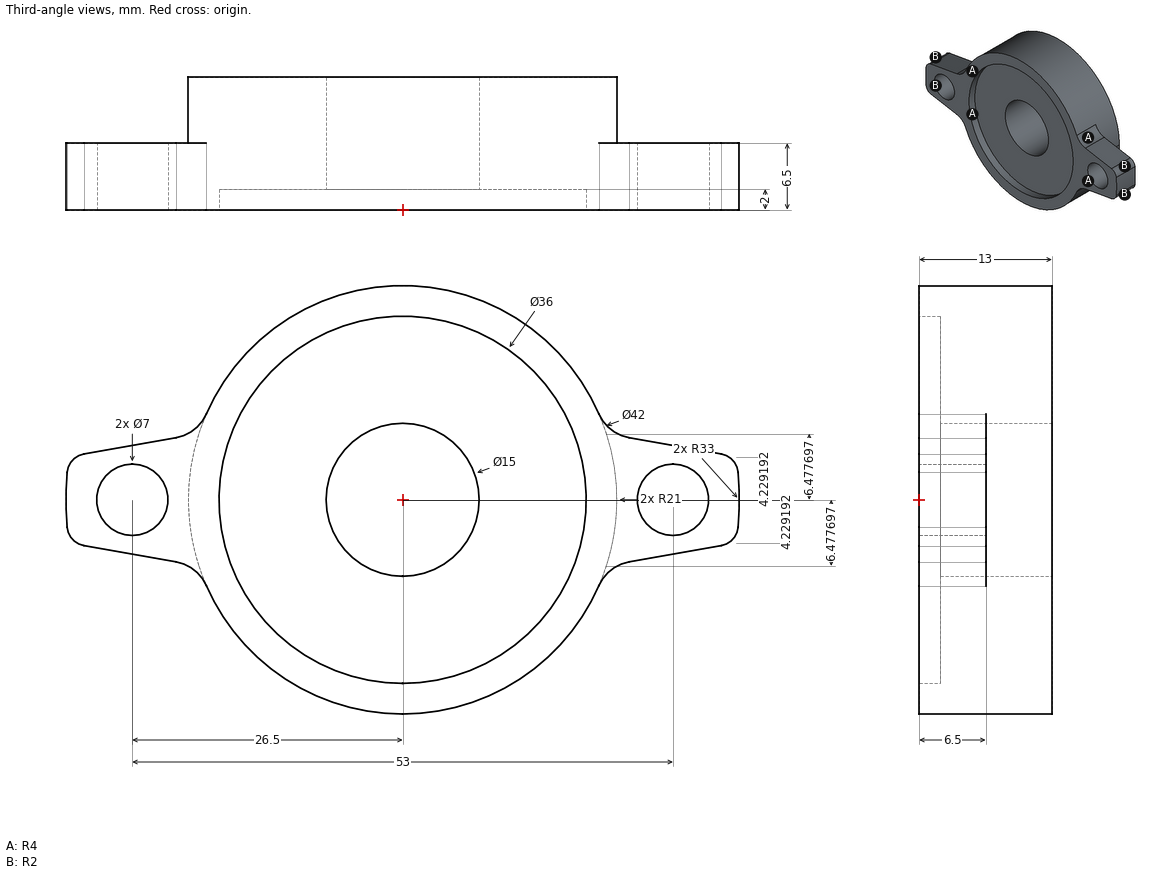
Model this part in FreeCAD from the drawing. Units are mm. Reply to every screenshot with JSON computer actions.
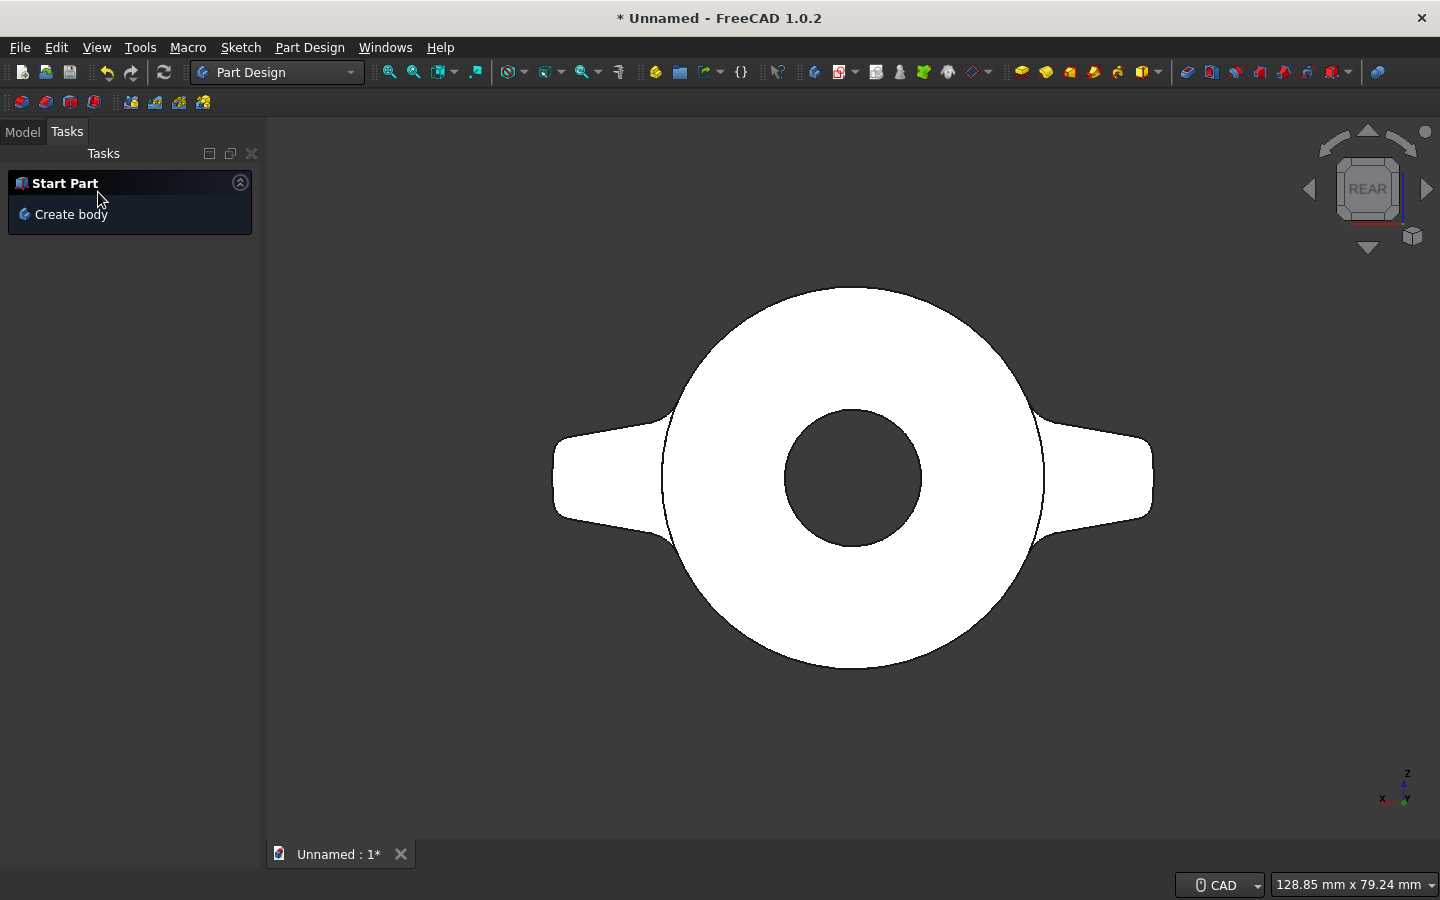
{"action": "left_click", "coordinate": [615, 477]}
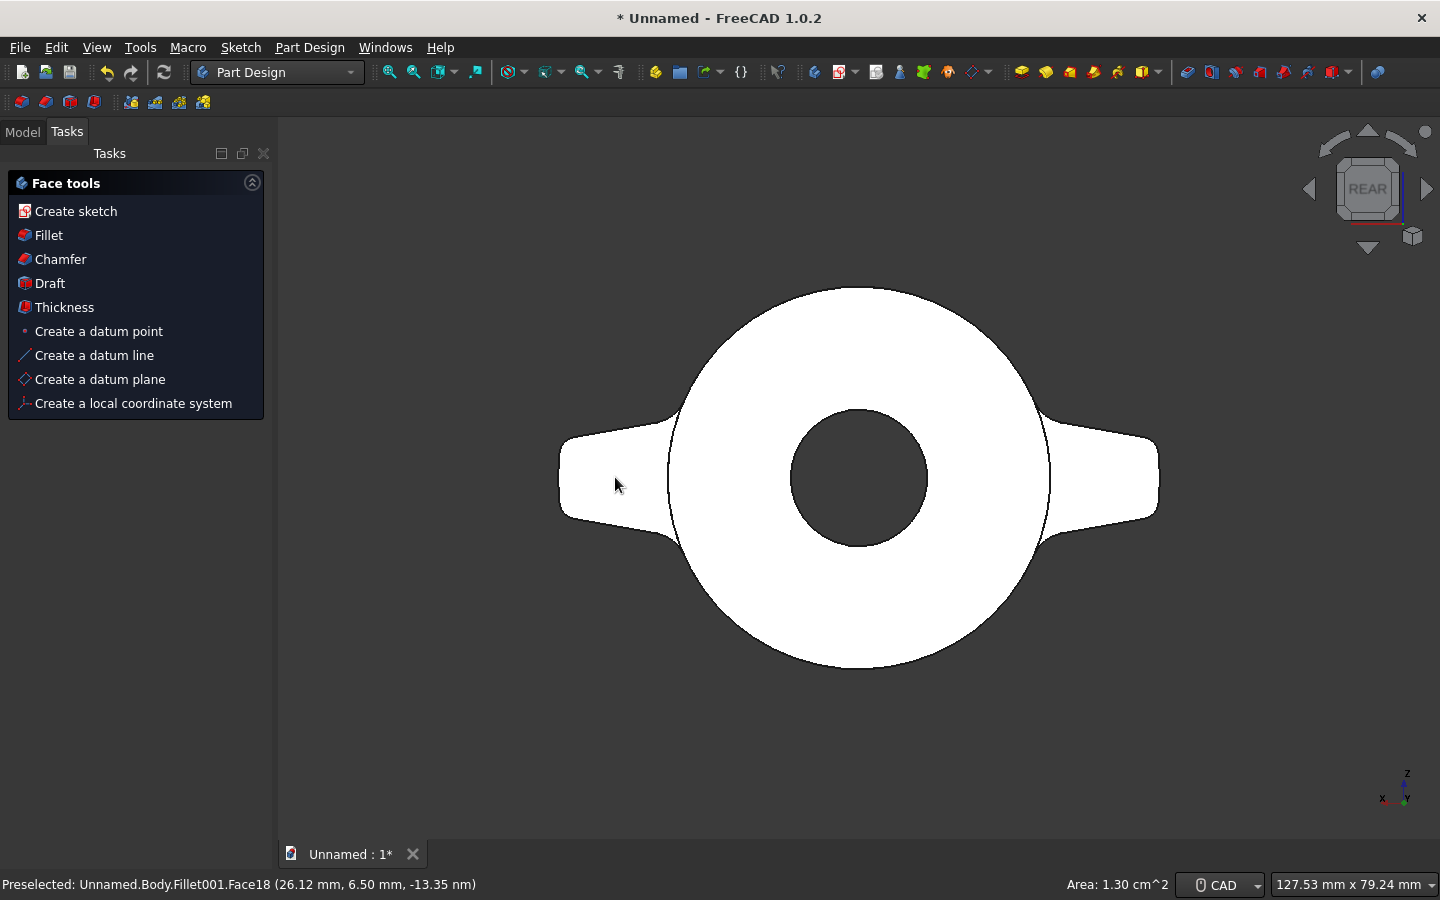
{"action": "left_click", "coordinate": [840, 72]}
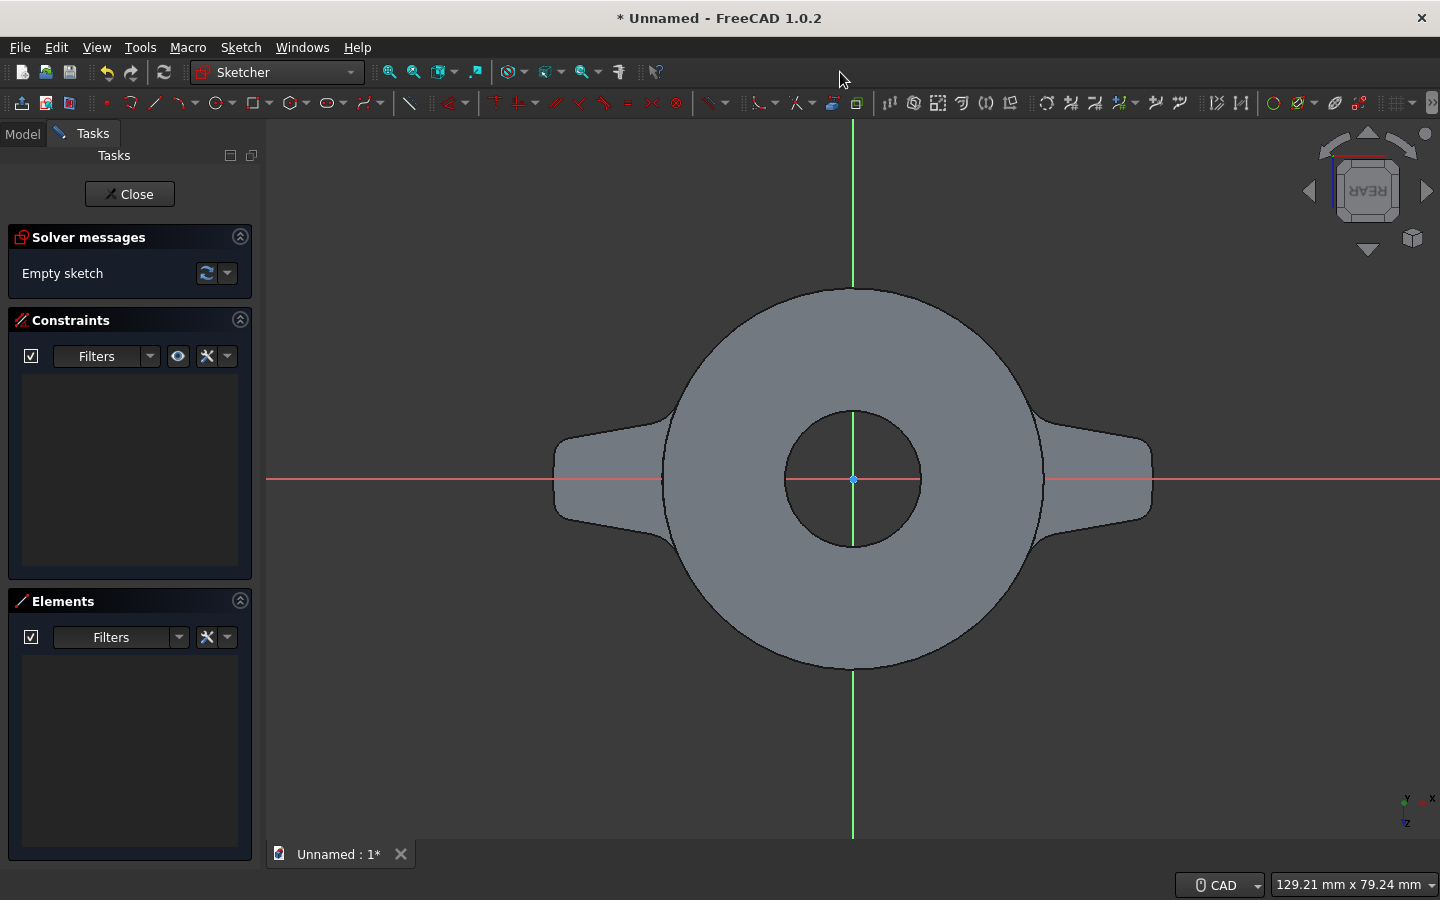
{"action": "left_click", "coordinate": [216, 104]}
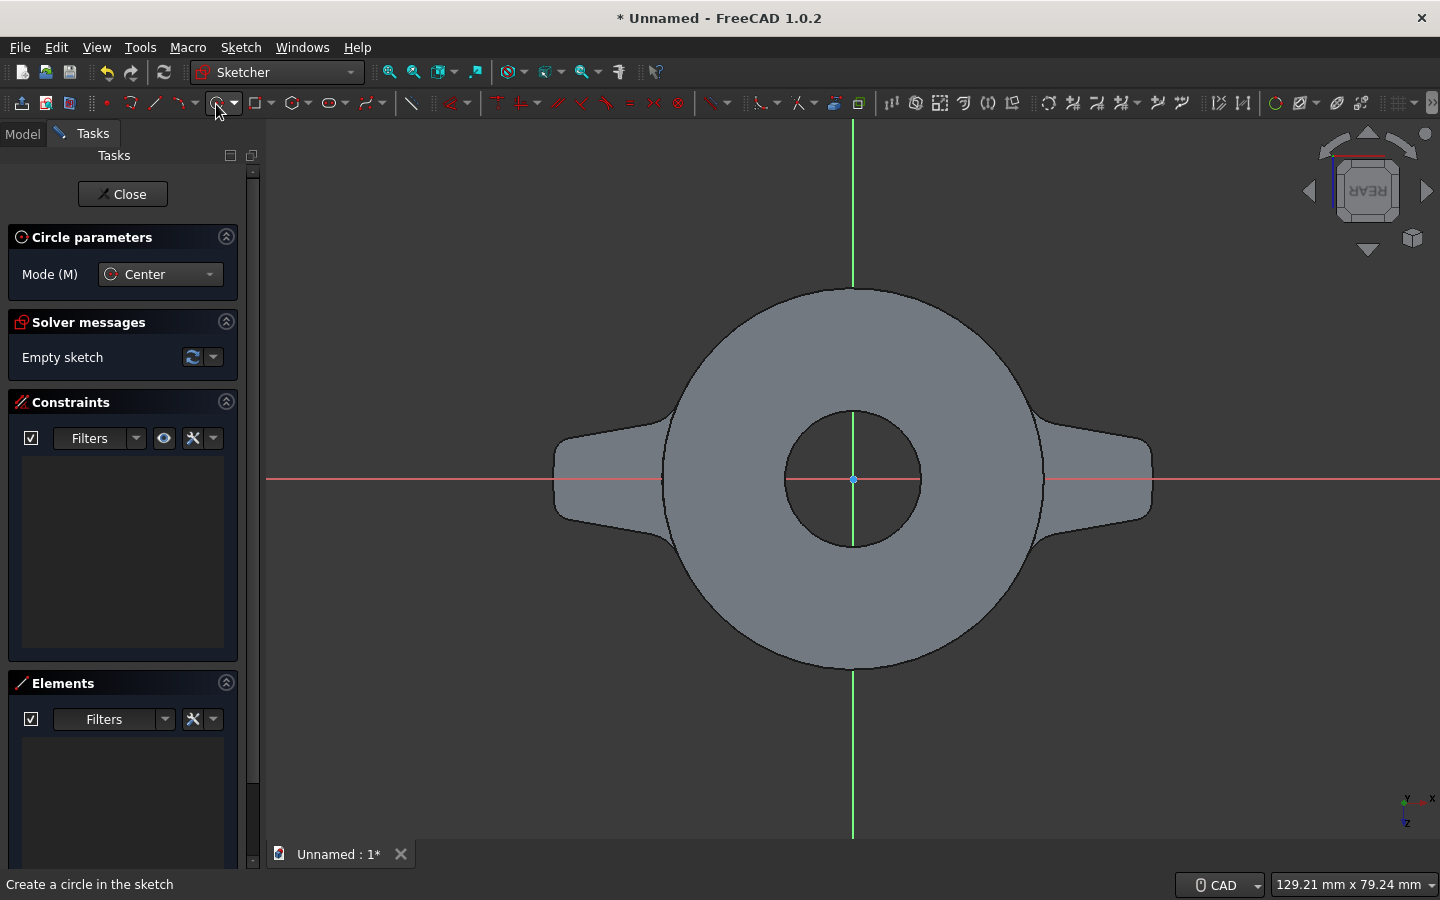
{"action": "left_click", "coordinate": [612, 479]}
{"action": "mouse_move", "coordinate": [635, 457]}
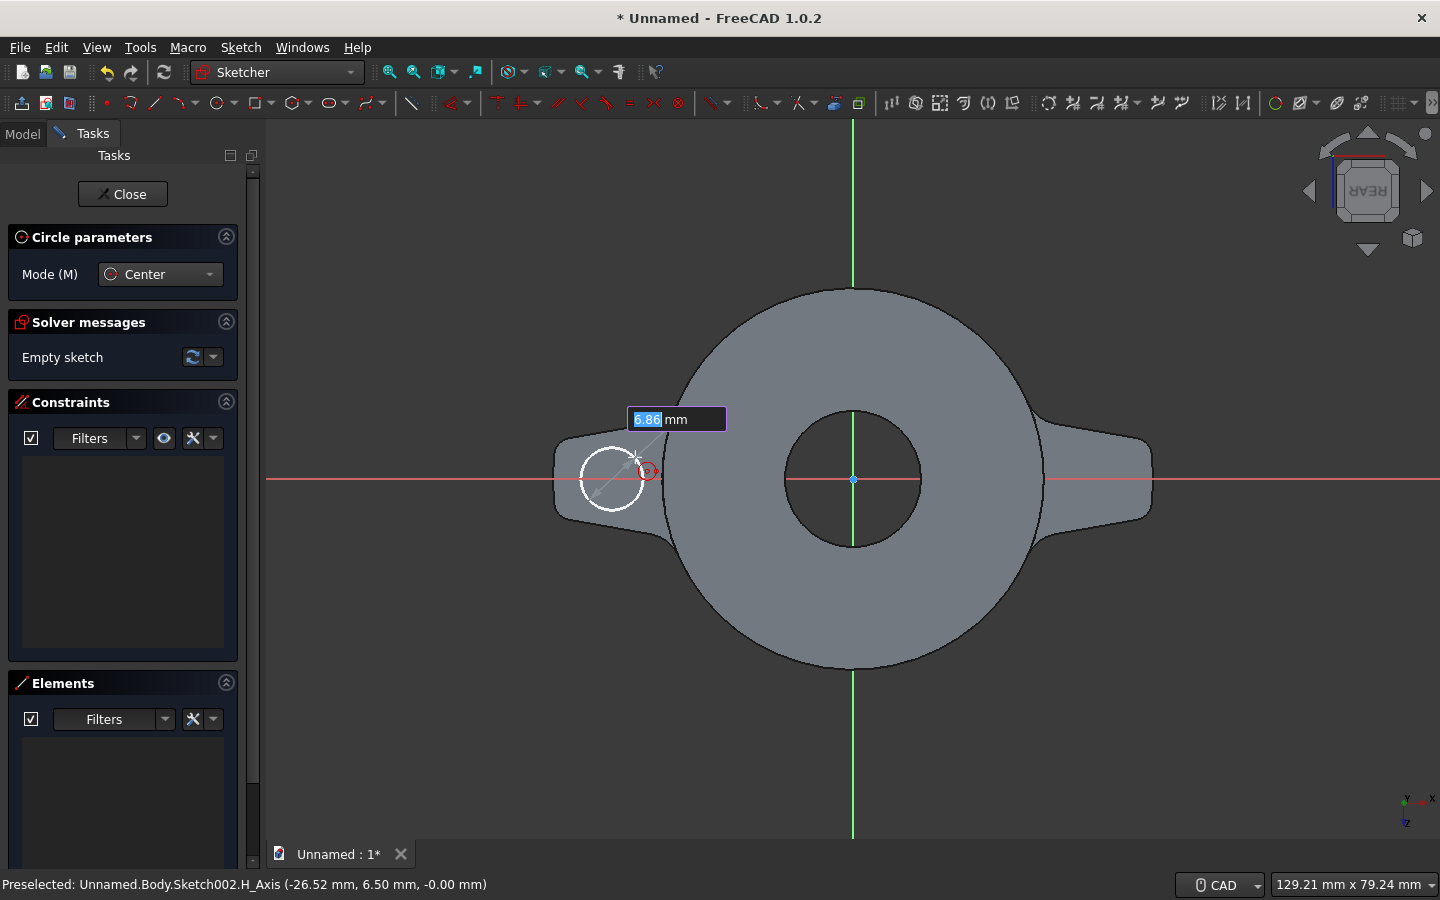
{"action": "type", "text": "7"}
{"action": "key", "text": "Return"}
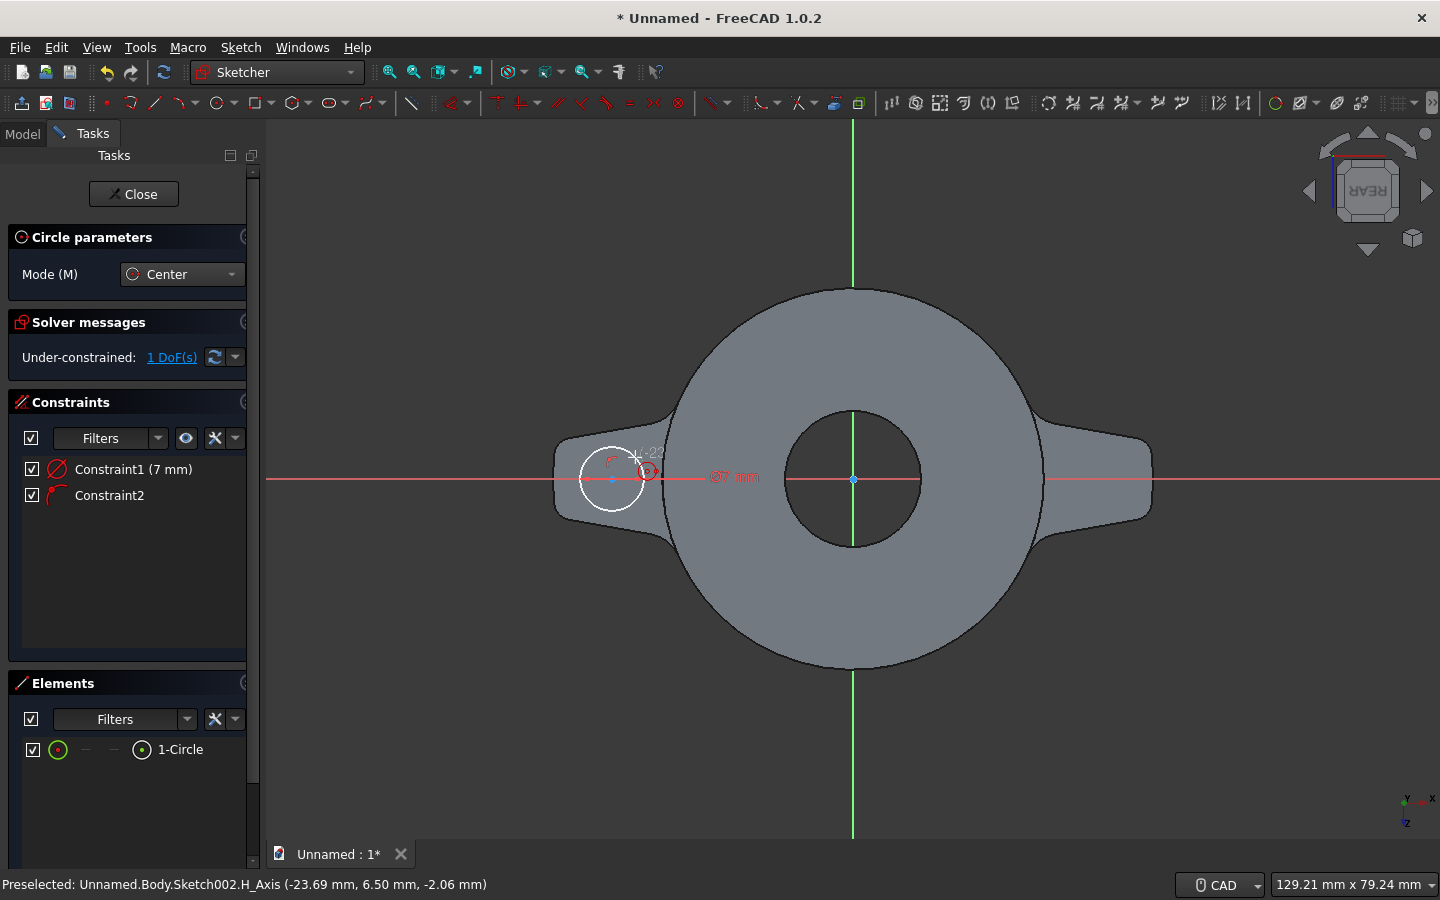
{"action": "left_click", "coordinate": [1094, 479]}
{"action": "mouse_move", "coordinate": [1116, 457]}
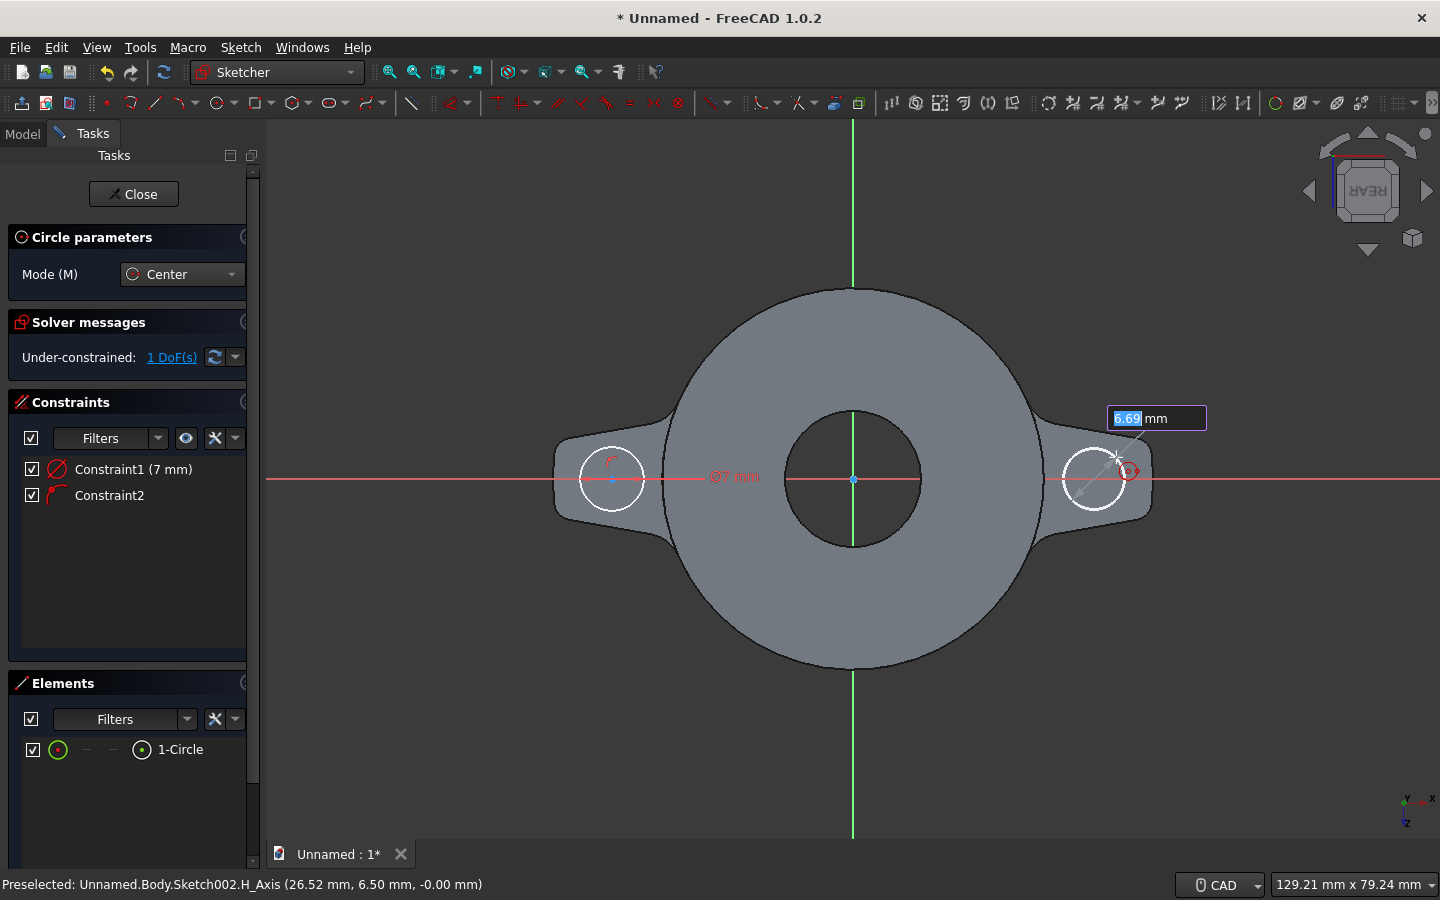
{"action": "type", "text": "7"}
{"action": "key", "text": "Return"}
{"action": "key", "text": "Escape"}